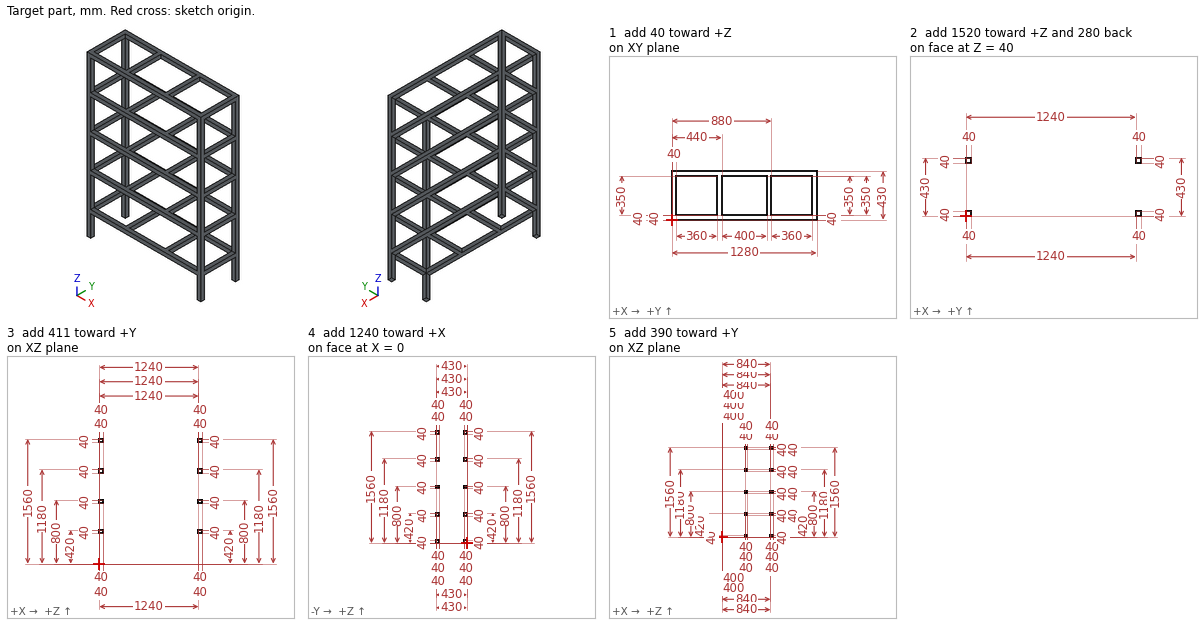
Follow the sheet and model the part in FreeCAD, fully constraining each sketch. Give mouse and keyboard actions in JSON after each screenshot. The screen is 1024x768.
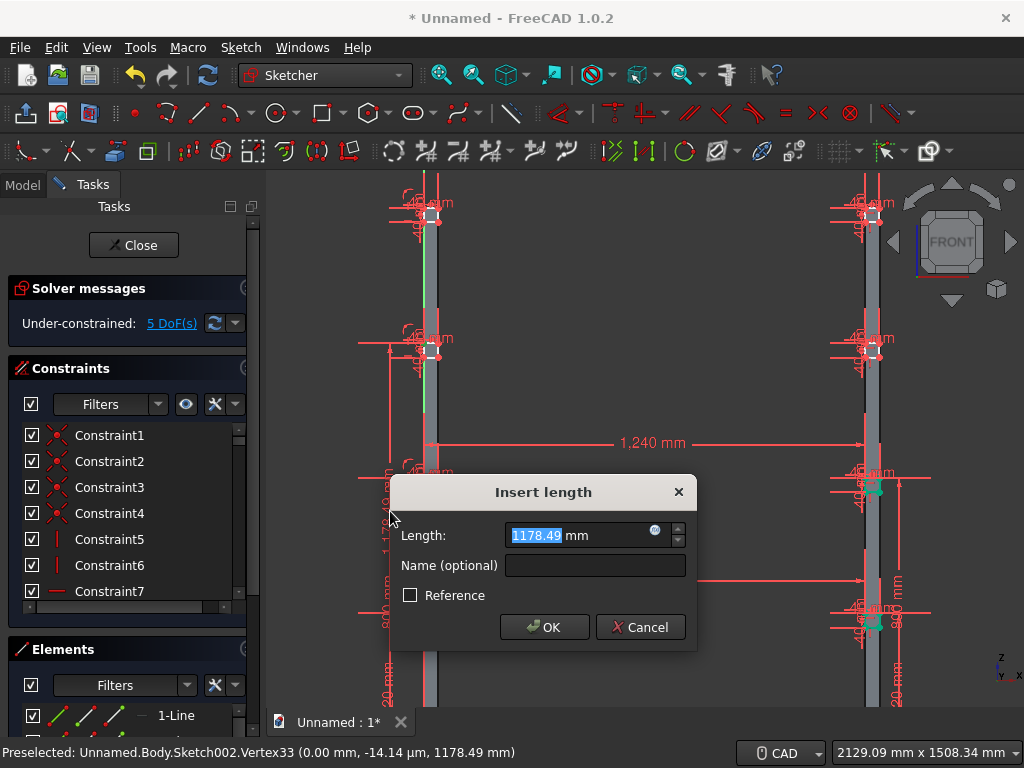
{"action": "type", "text": "1180"}
{"action": "key", "text": "Return"}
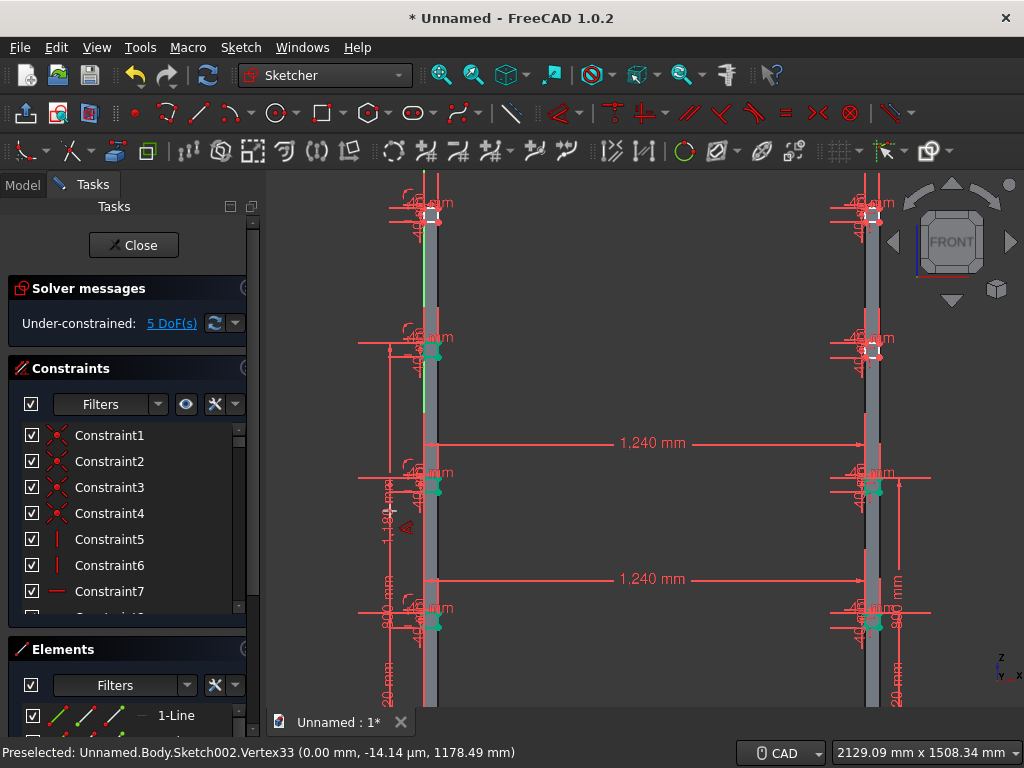
{"action": "scroll", "coordinate": [423, 343], "scroll_direction": "down", "scroll_amount": 2}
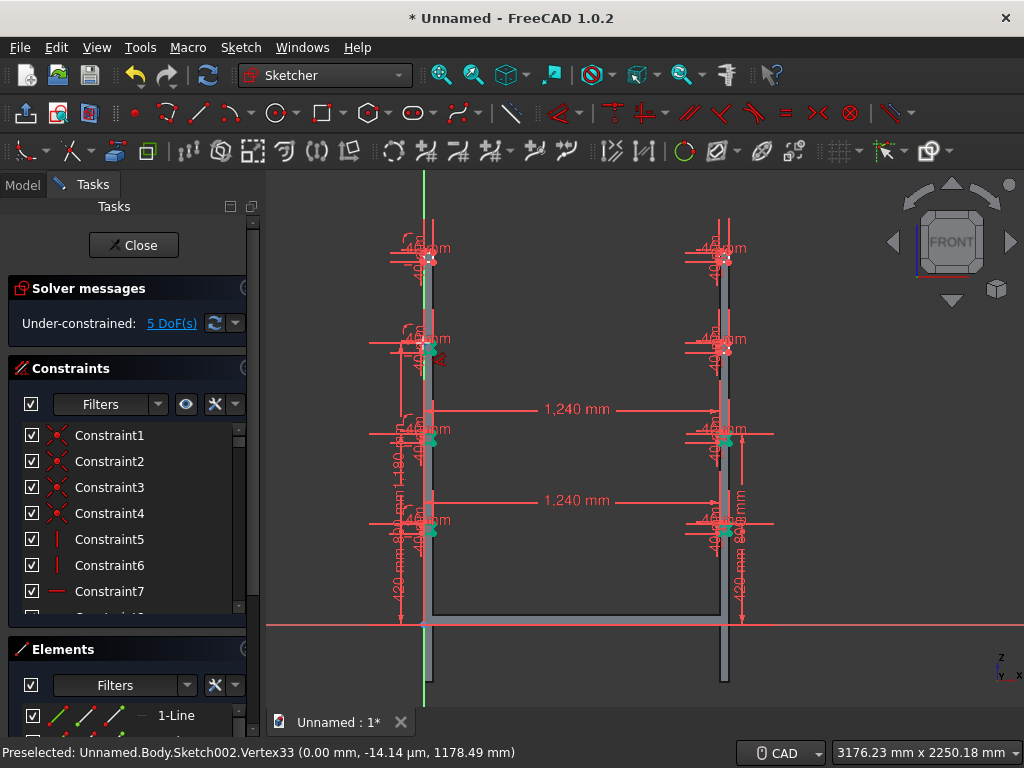
{"action": "scroll", "coordinate": [719, 343], "scroll_direction": "up", "scroll_amount": 2}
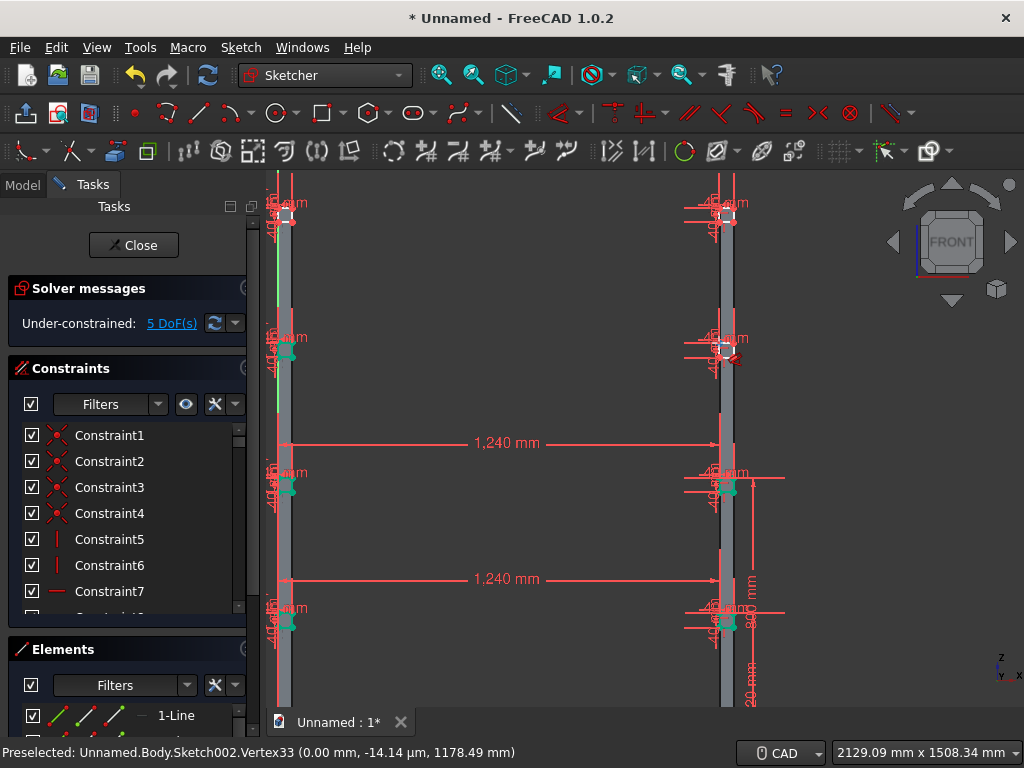
{"action": "left_click", "coordinate": [719, 343]}
{"action": "left_click", "coordinate": [507, 309]}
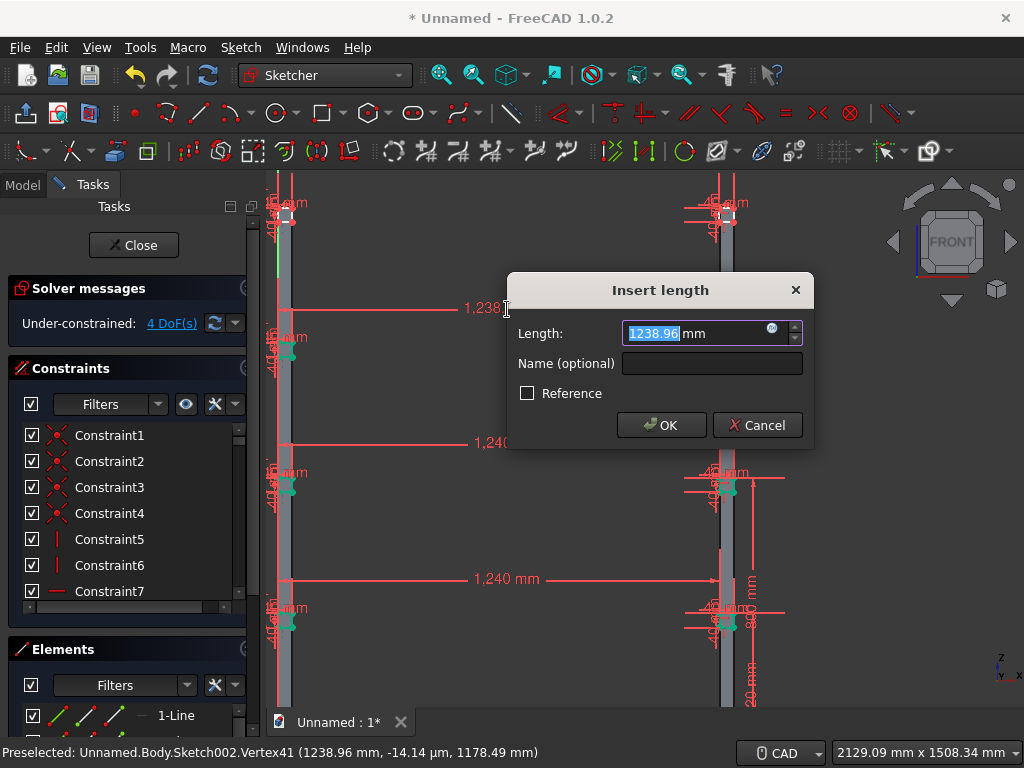
{"action": "type", "text": "1240"}
{"action": "key", "text": "Return"}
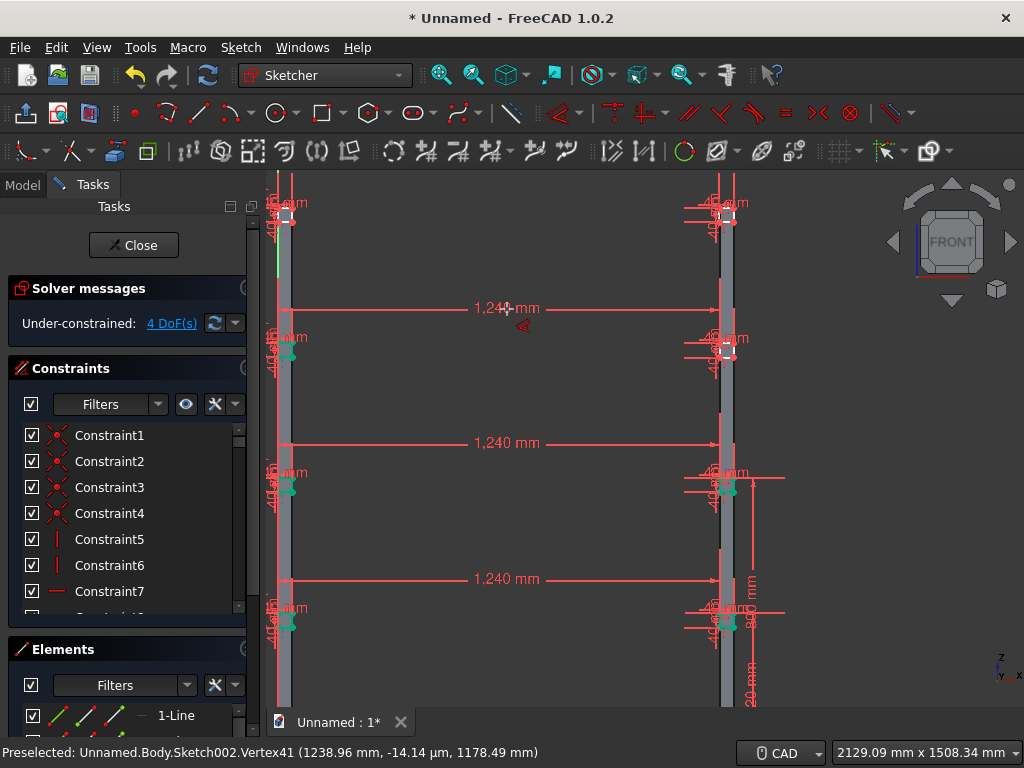
{"action": "left_click", "coordinate": [720, 343]}
{"action": "left_click", "coordinate": [754, 511]}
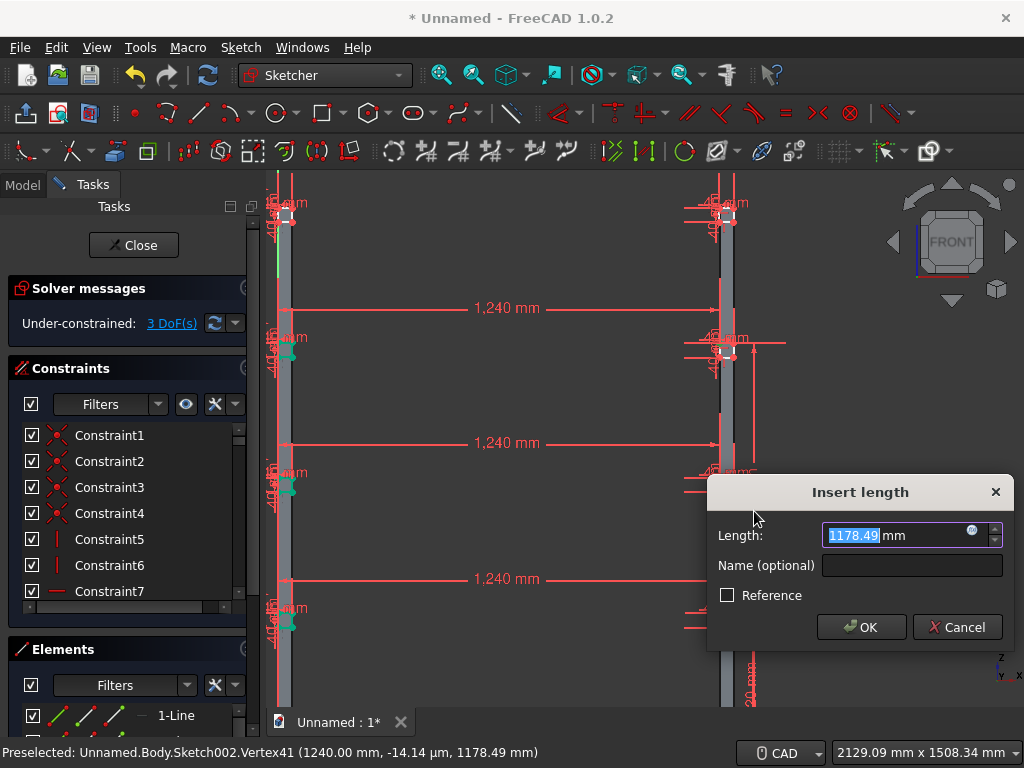
{"action": "type", "text": "1180"}
{"action": "key", "text": "Return"}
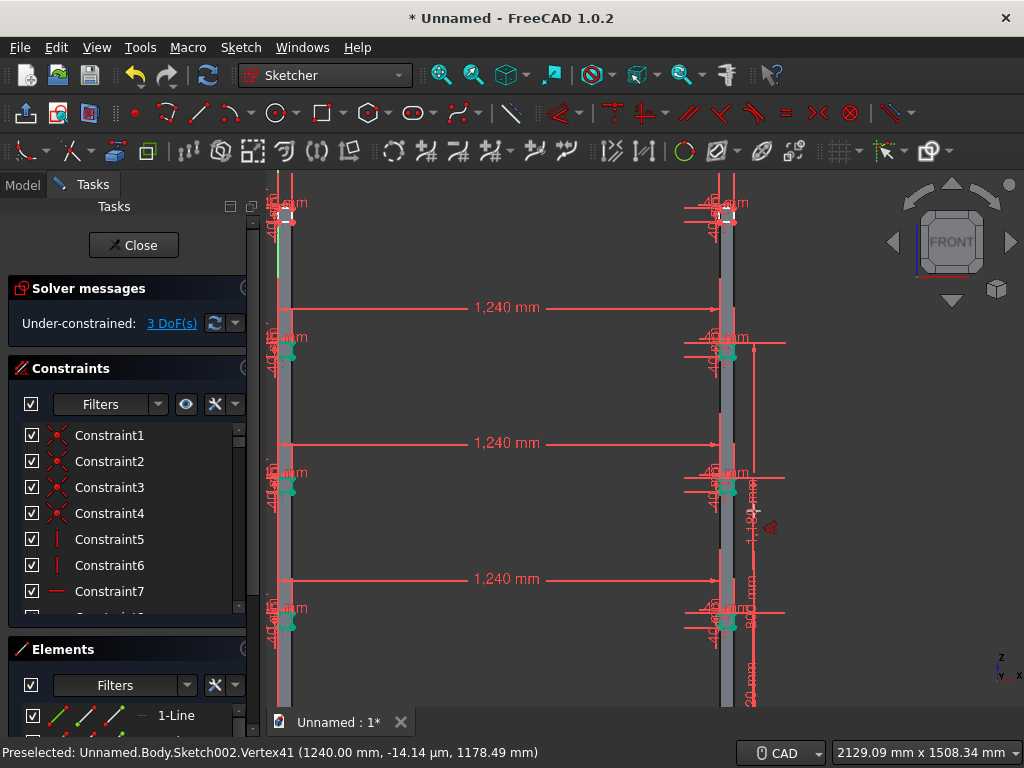
{"action": "scroll", "coordinate": [720, 343], "scroll_direction": "down", "scroll_amount": 2}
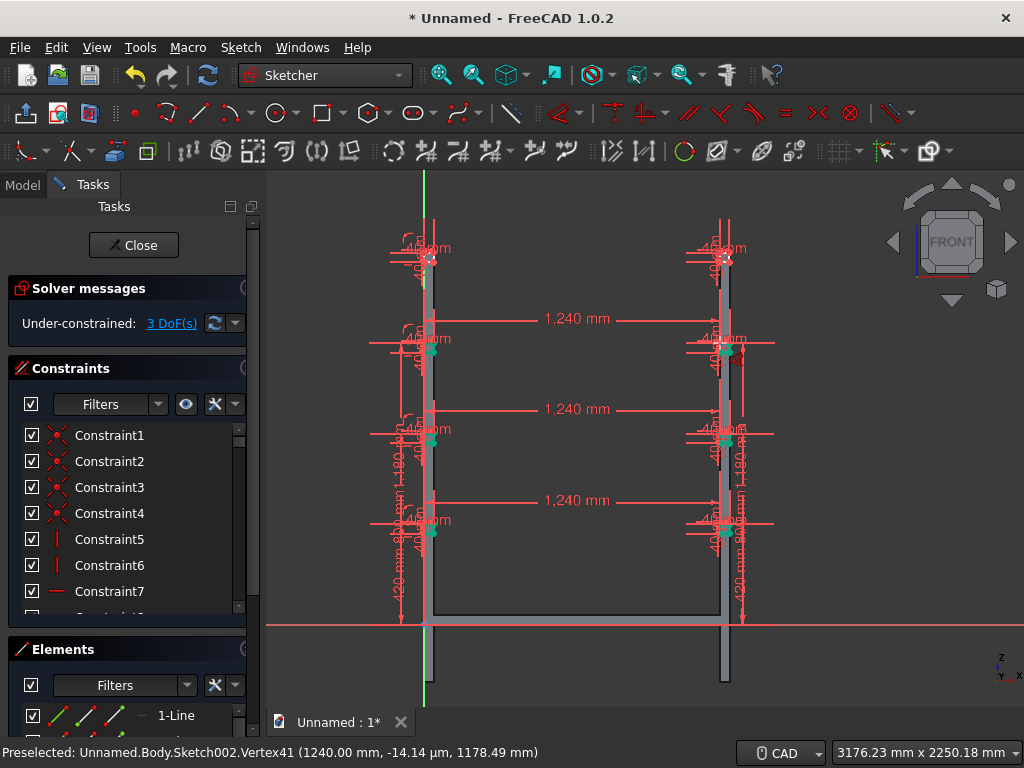
{"action": "scroll", "coordinate": [424, 253], "scroll_direction": "up", "scroll_amount": 2}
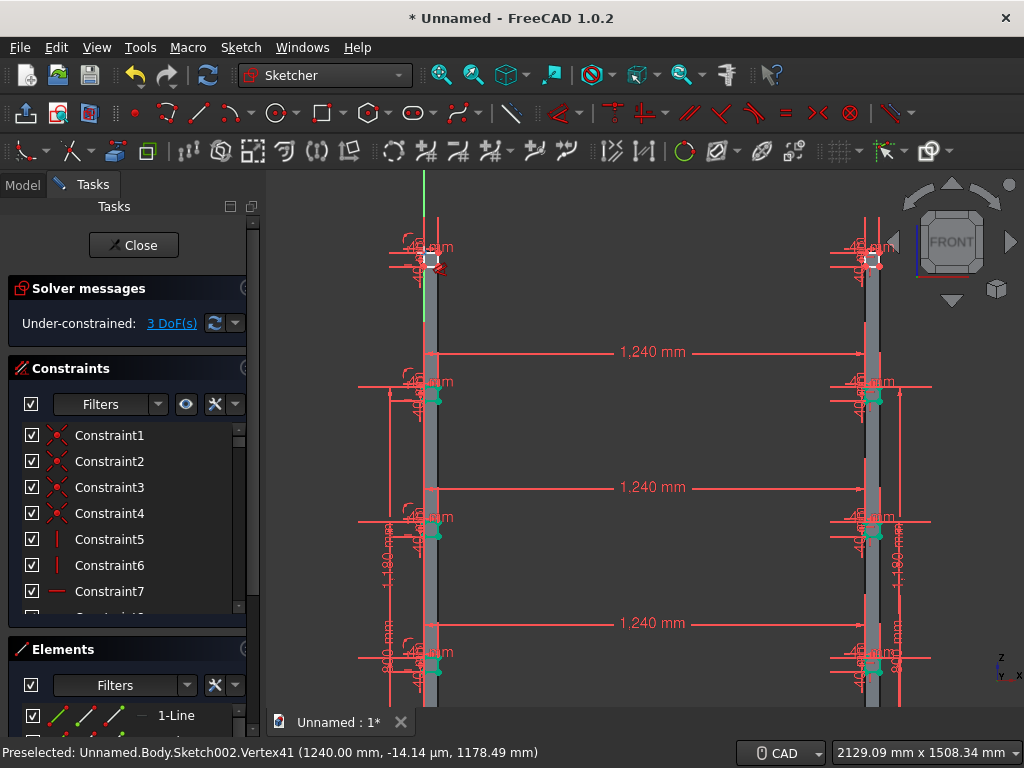
{"action": "left_click", "coordinate": [424, 253]}
{"action": "left_click", "coordinate": [390, 466]}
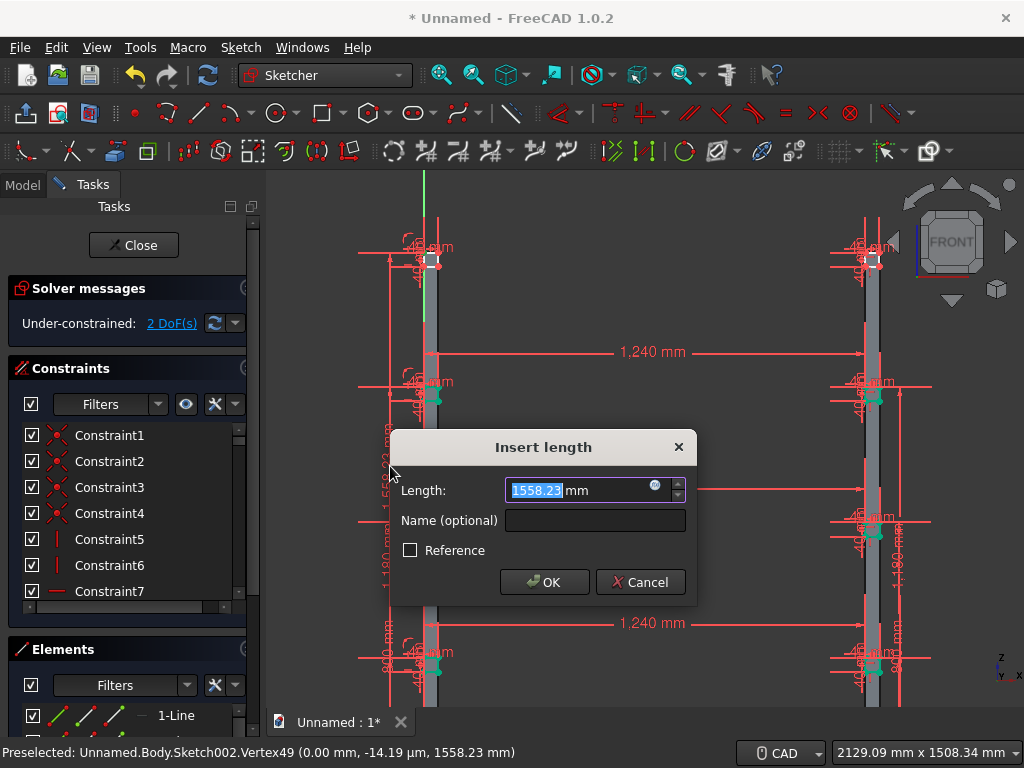
{"action": "type", "text": "1560"}
{"action": "key", "text": "Return"}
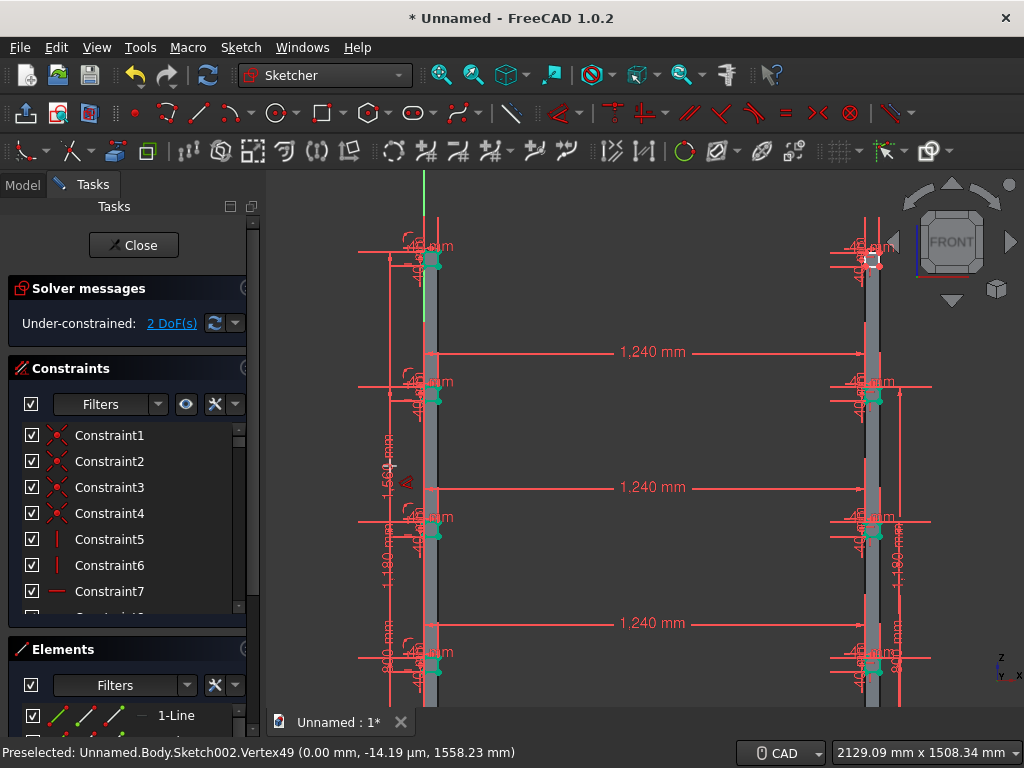
{"action": "scroll", "coordinate": [423, 253], "scroll_direction": "down", "scroll_amount": 2}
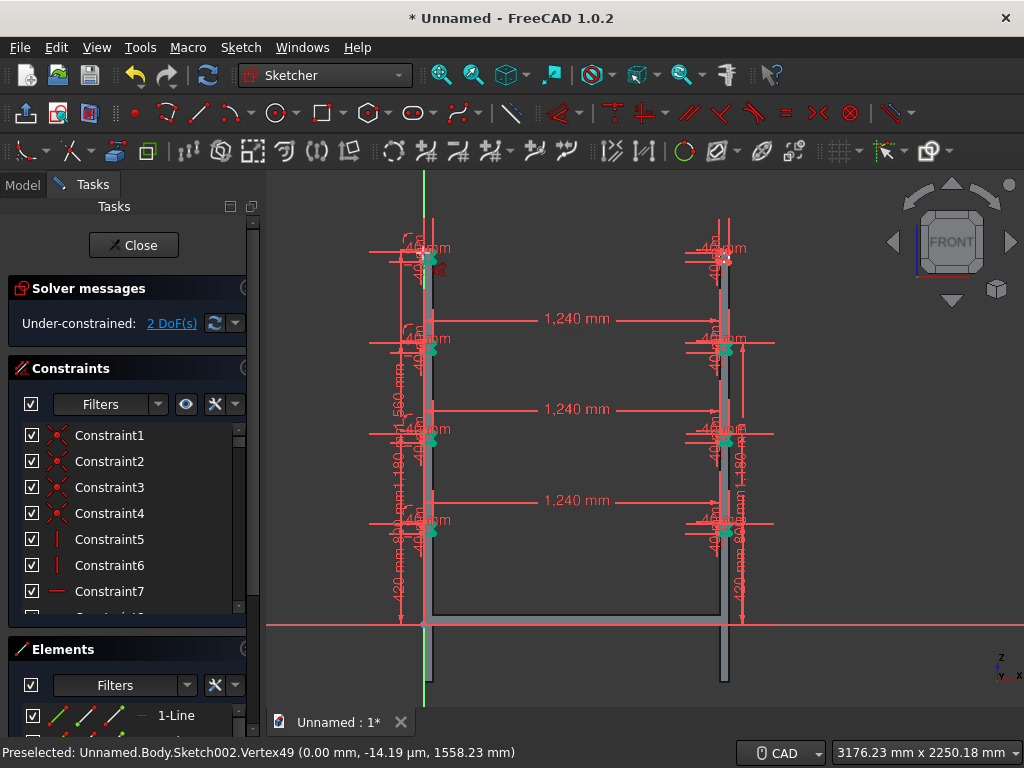
{"action": "scroll", "coordinate": [719, 253], "scroll_direction": "up", "scroll_amount": 2}